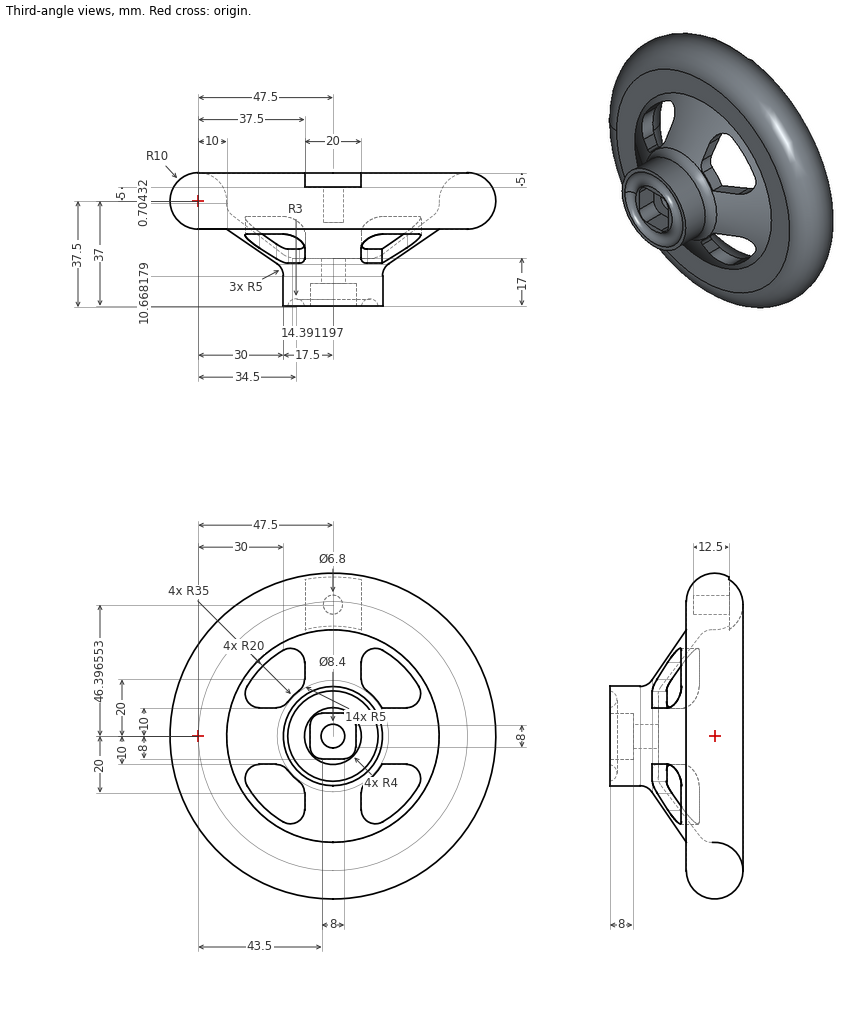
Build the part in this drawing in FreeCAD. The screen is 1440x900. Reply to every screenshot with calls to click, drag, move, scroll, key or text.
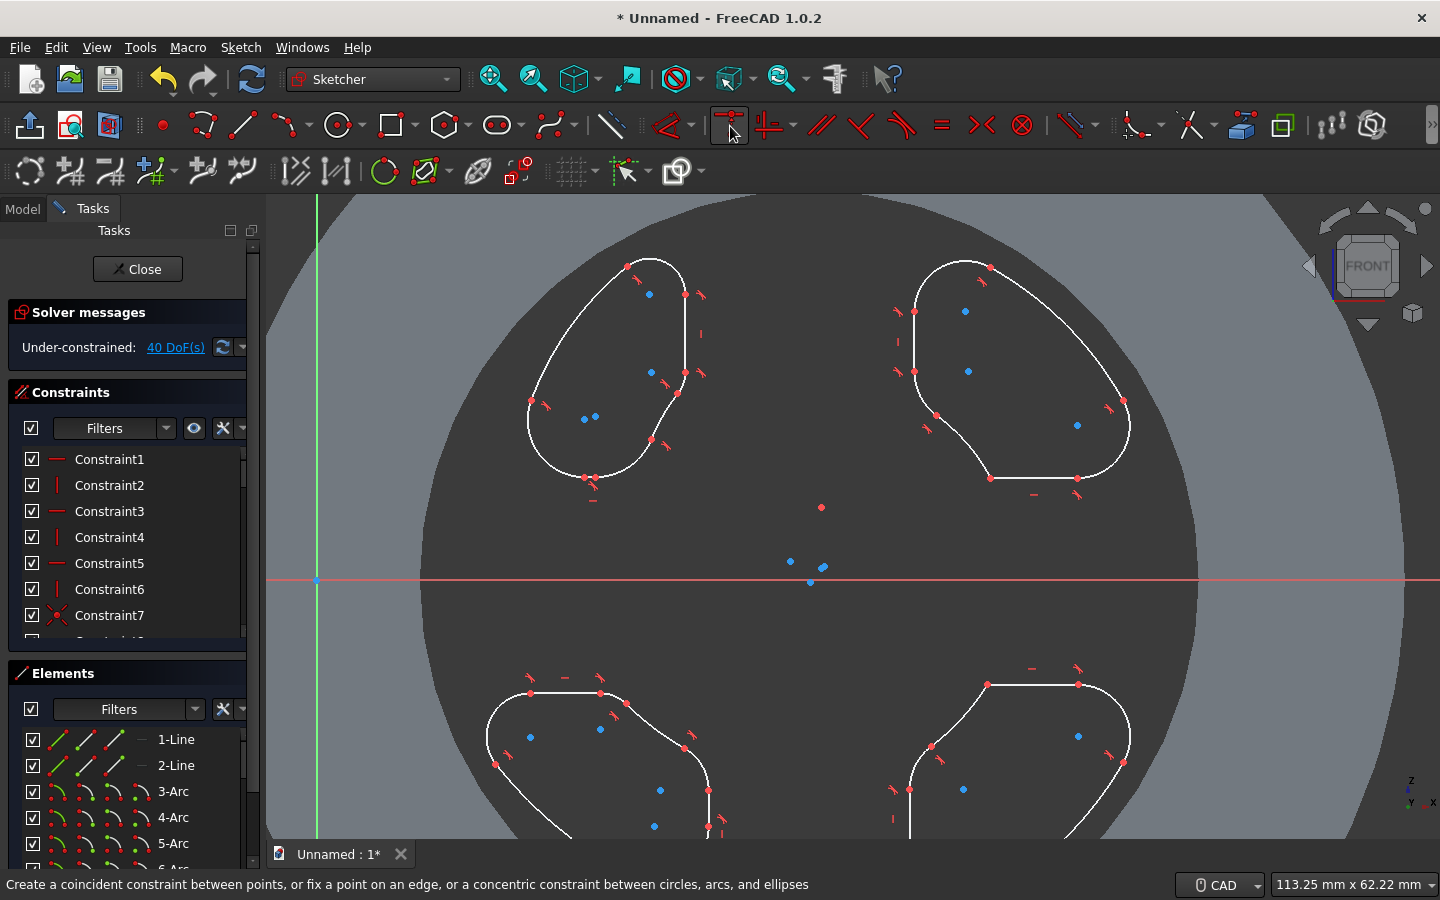
click(591, 301)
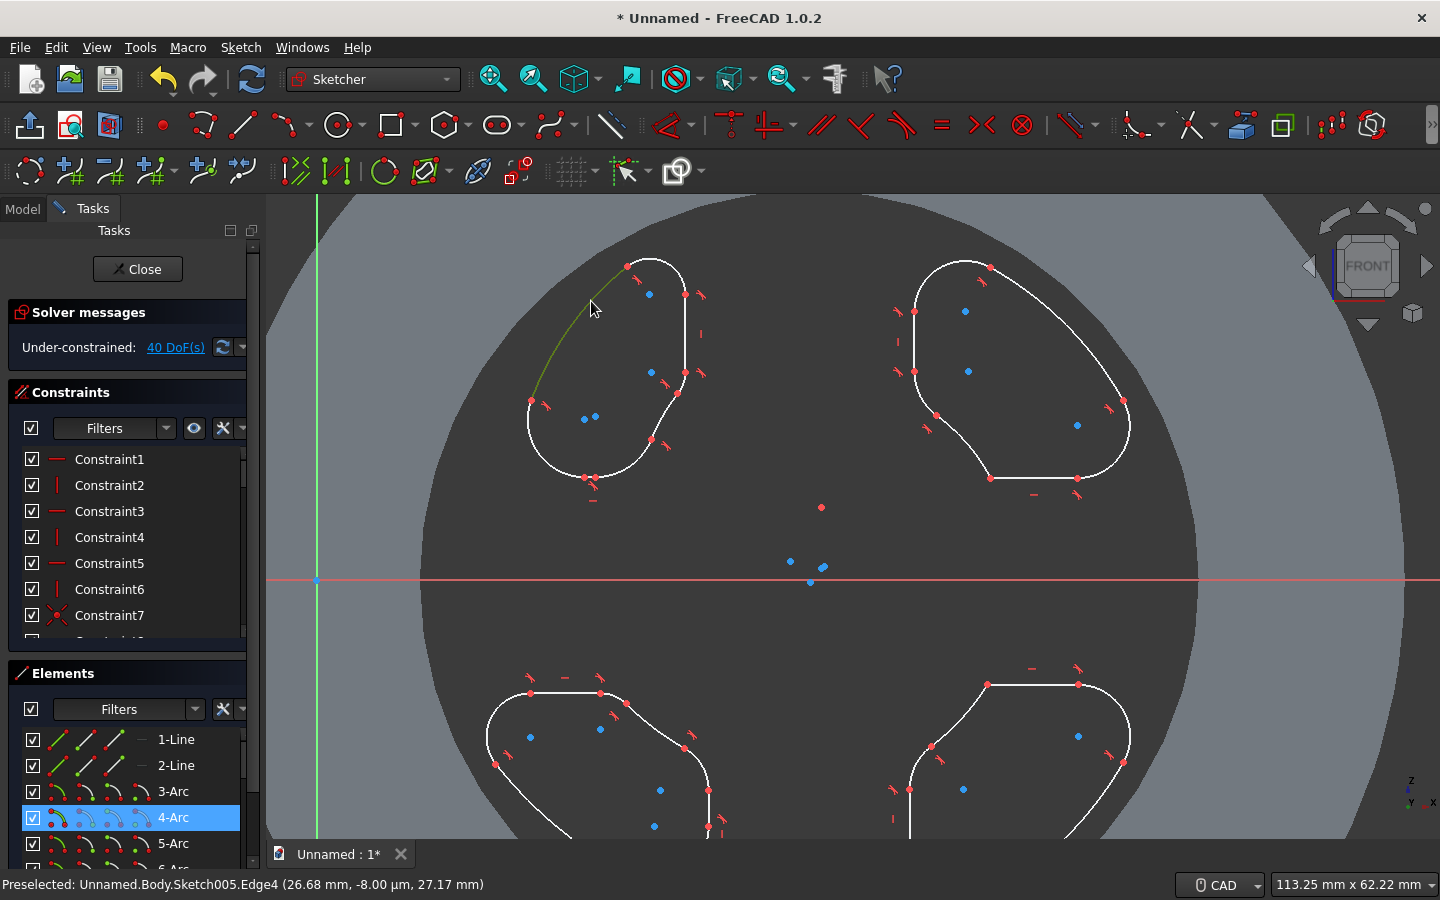
click(1091, 809)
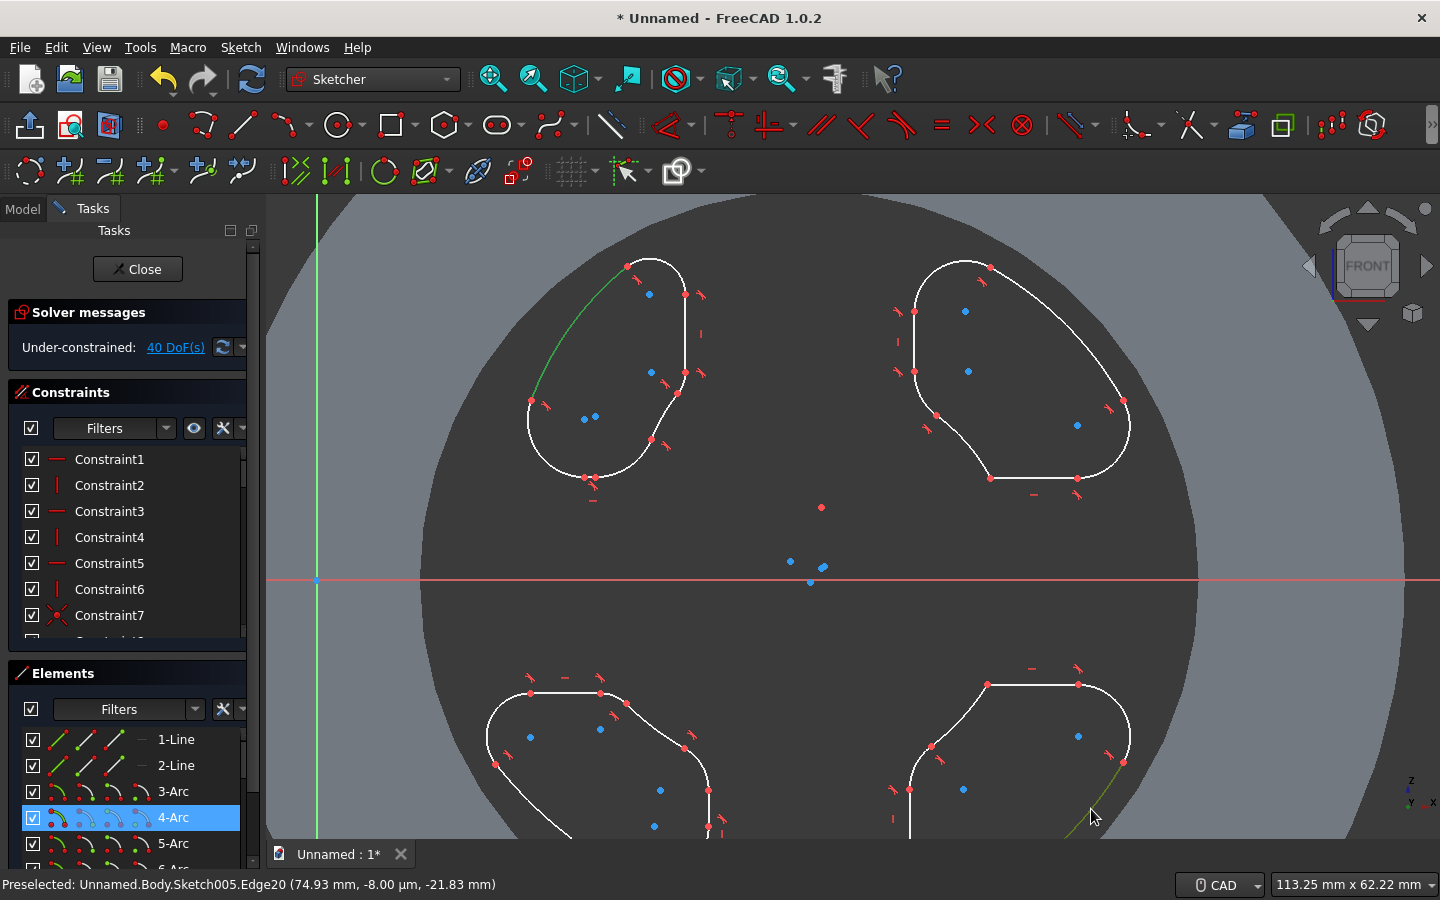
click(730, 126)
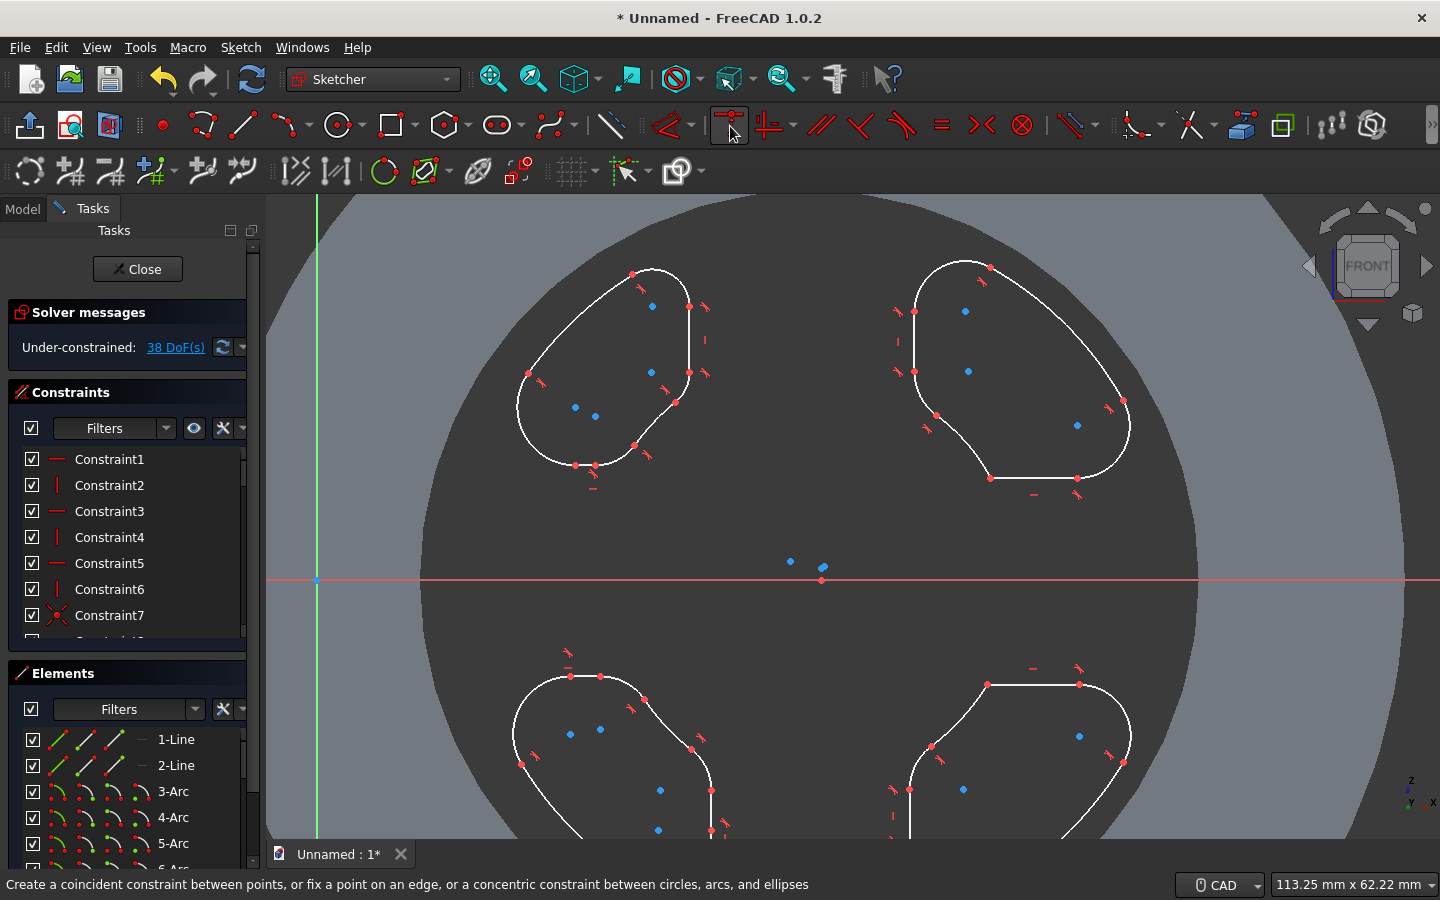
click(597, 300)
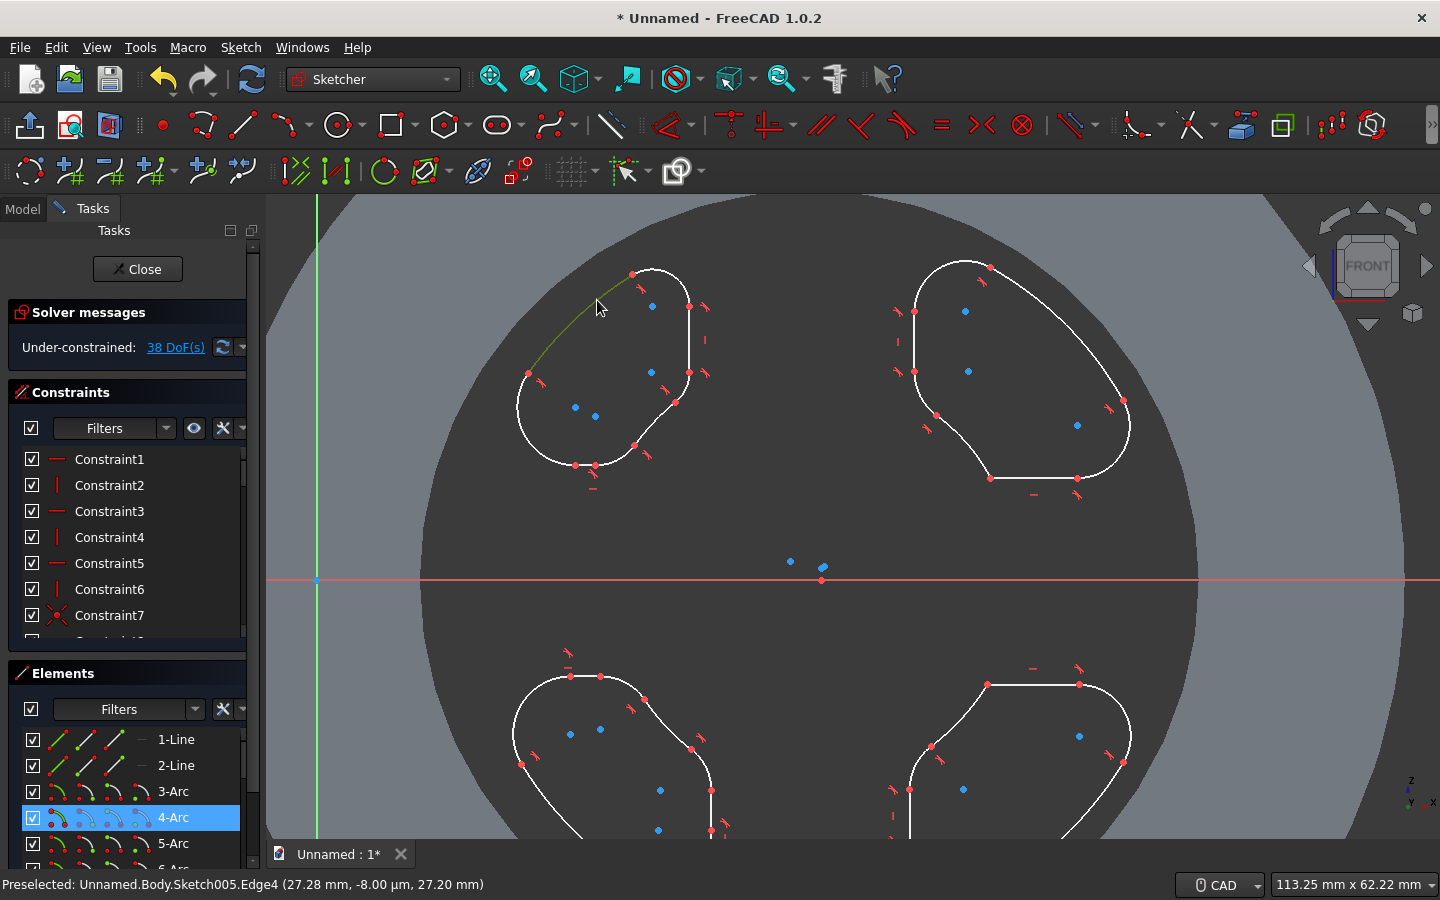
click(950, 730)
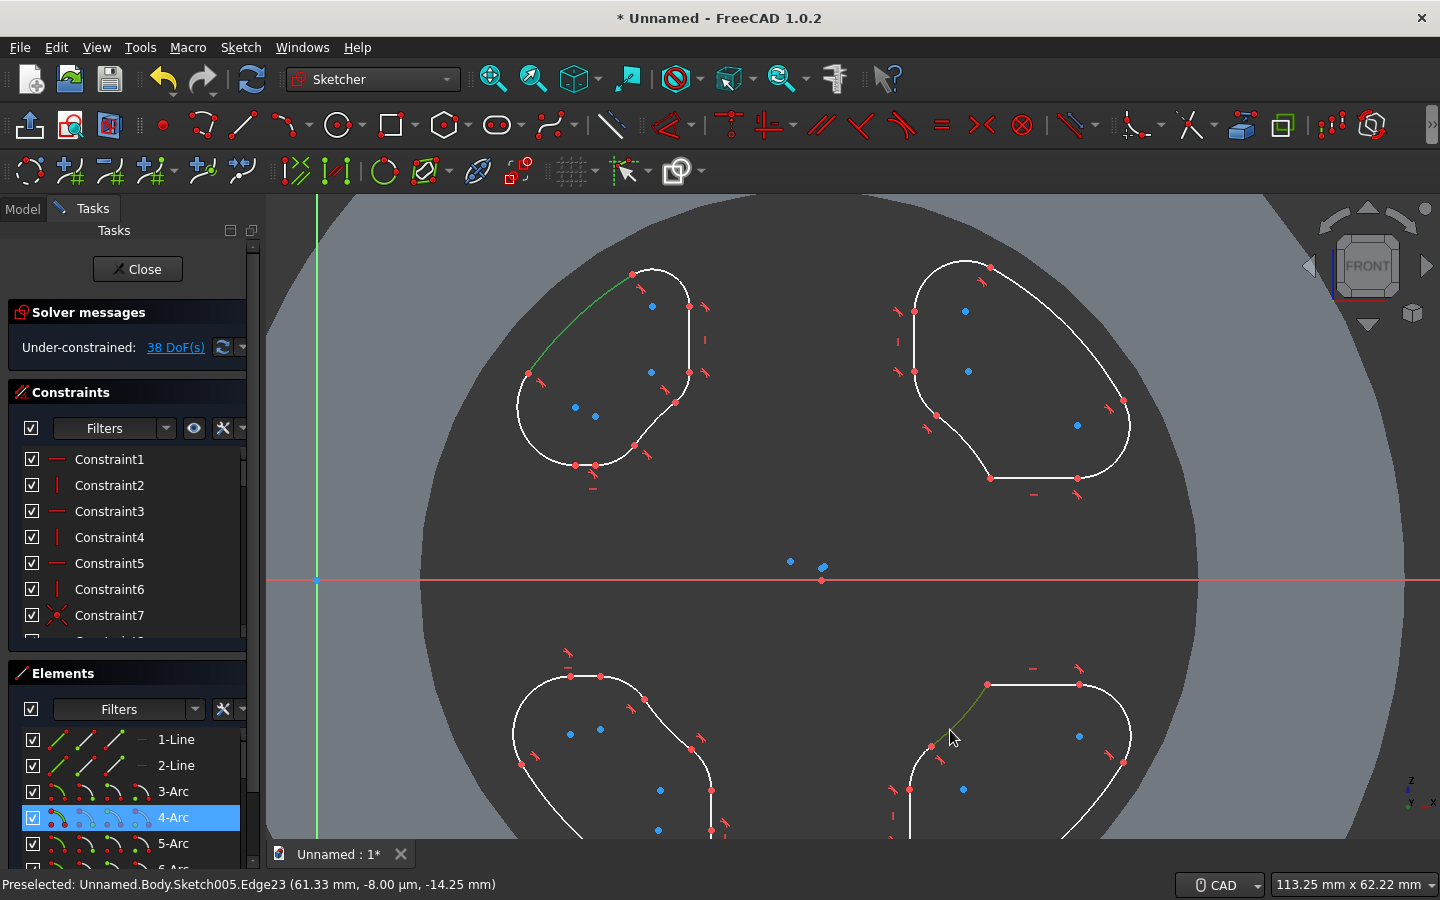
click(730, 126)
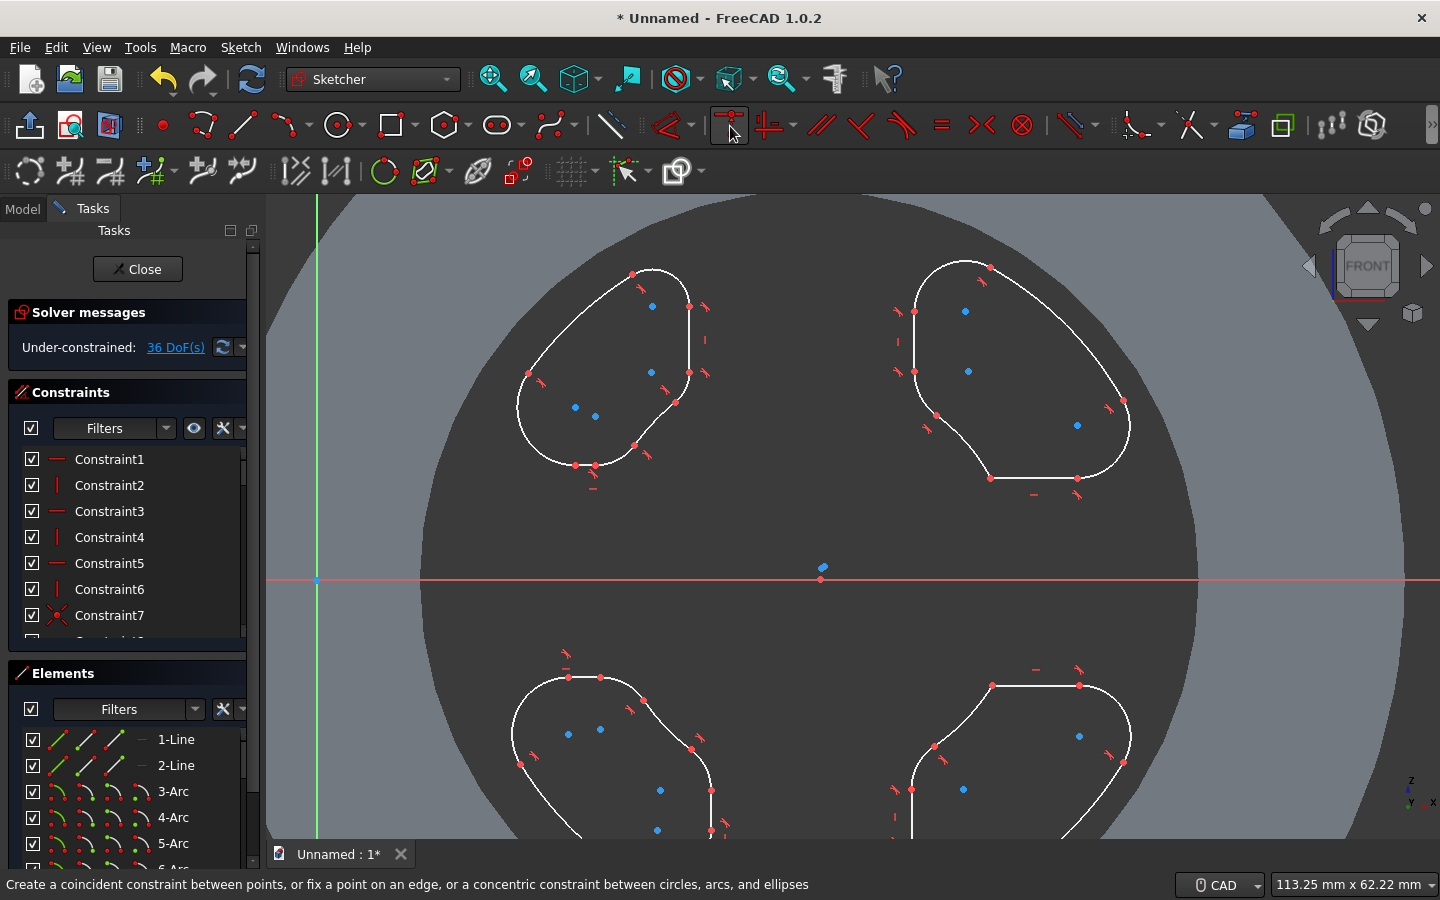
click(597, 300)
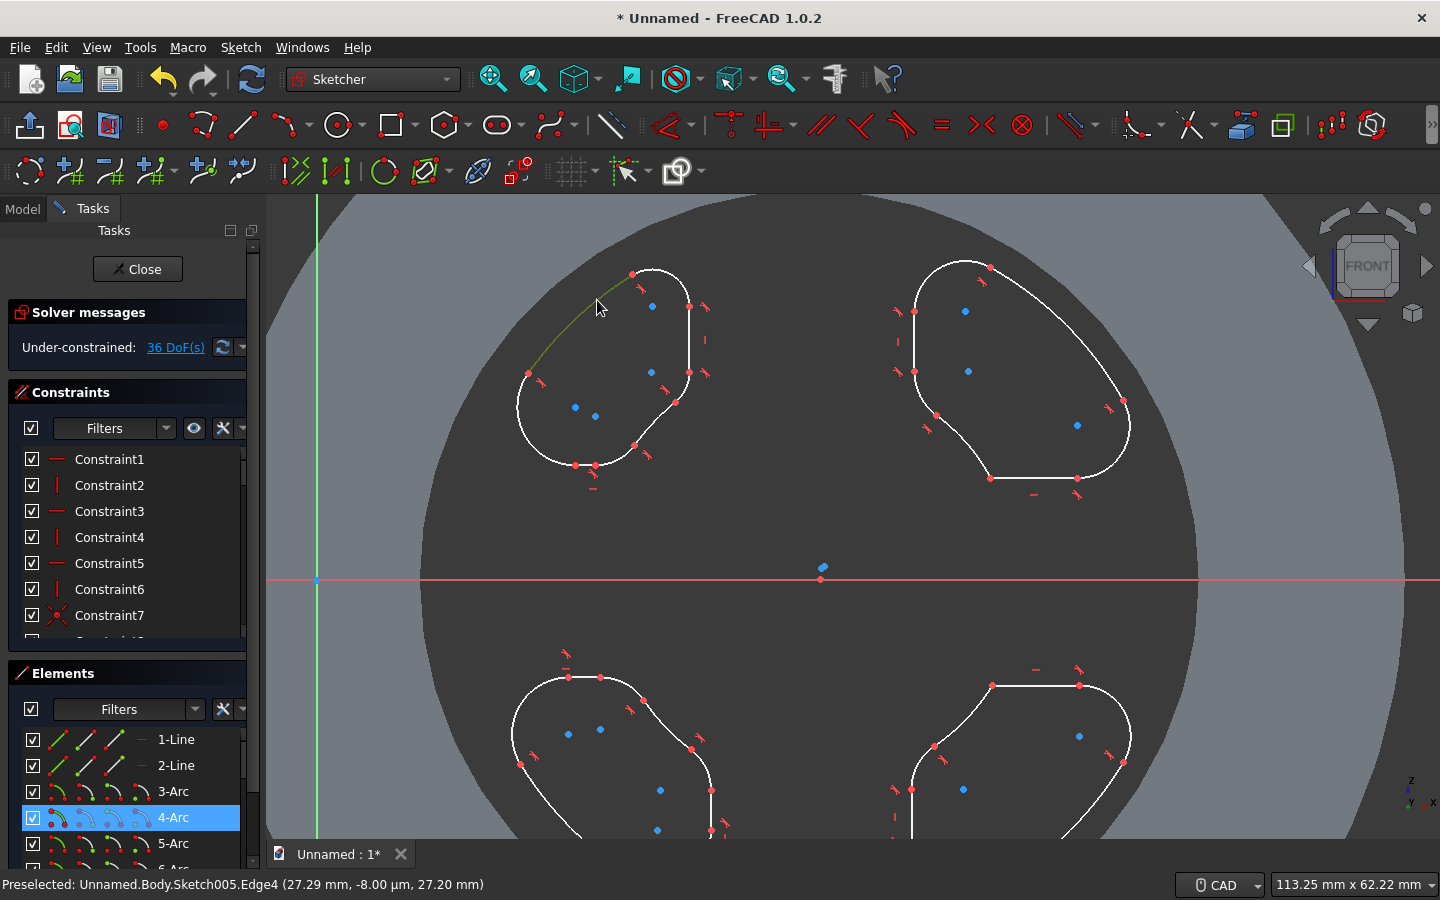
click(978, 457)